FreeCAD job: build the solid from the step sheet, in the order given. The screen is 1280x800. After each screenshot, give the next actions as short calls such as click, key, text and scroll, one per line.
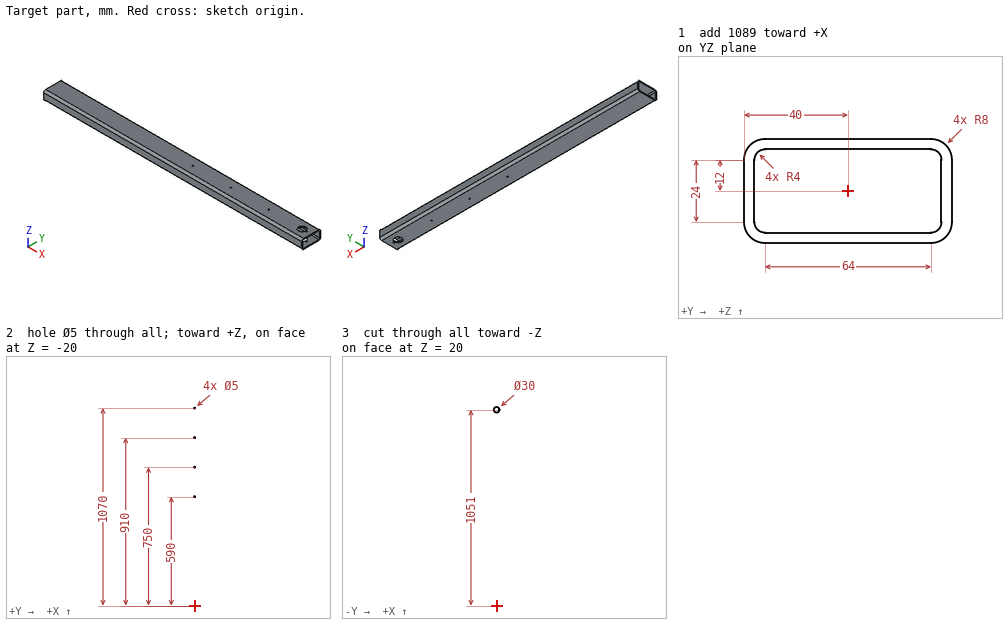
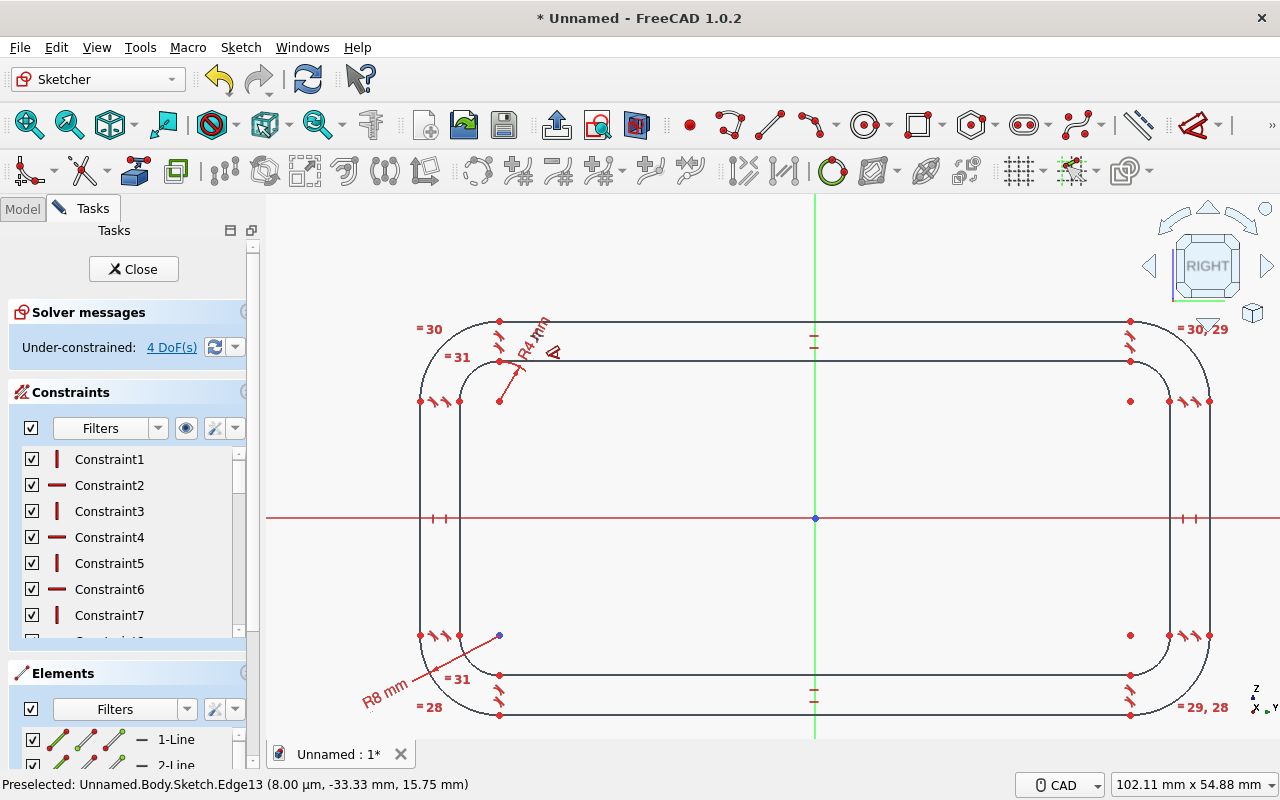
click(420, 471)
click(386, 464)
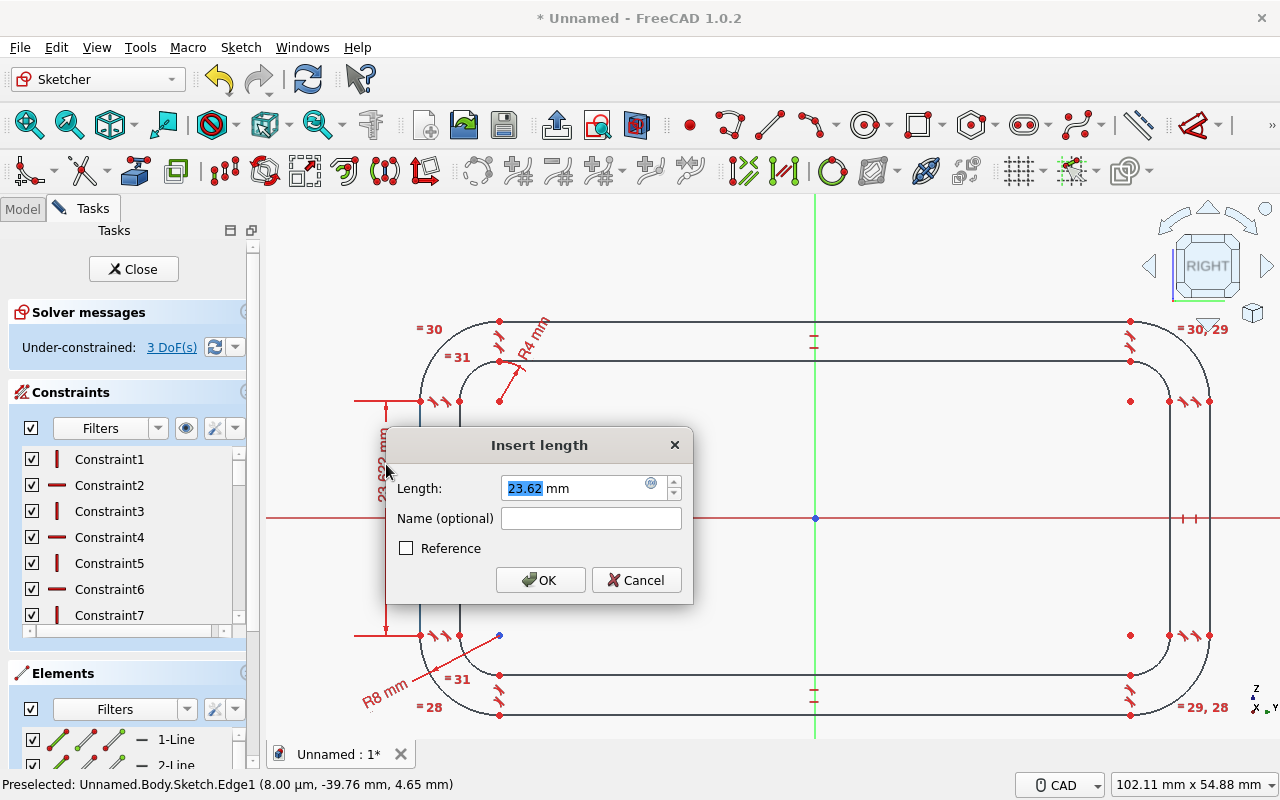
text(24)
key(Return)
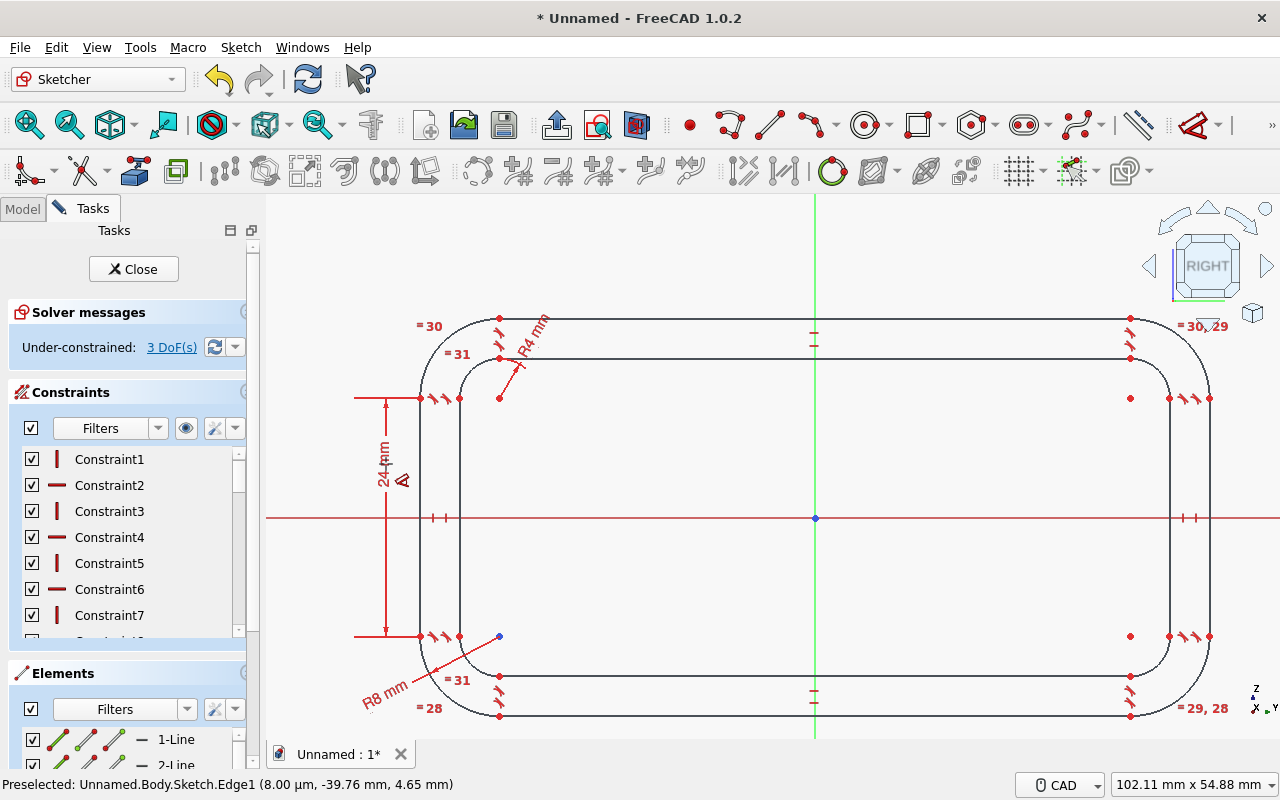
scroll(480, 361, down, 2)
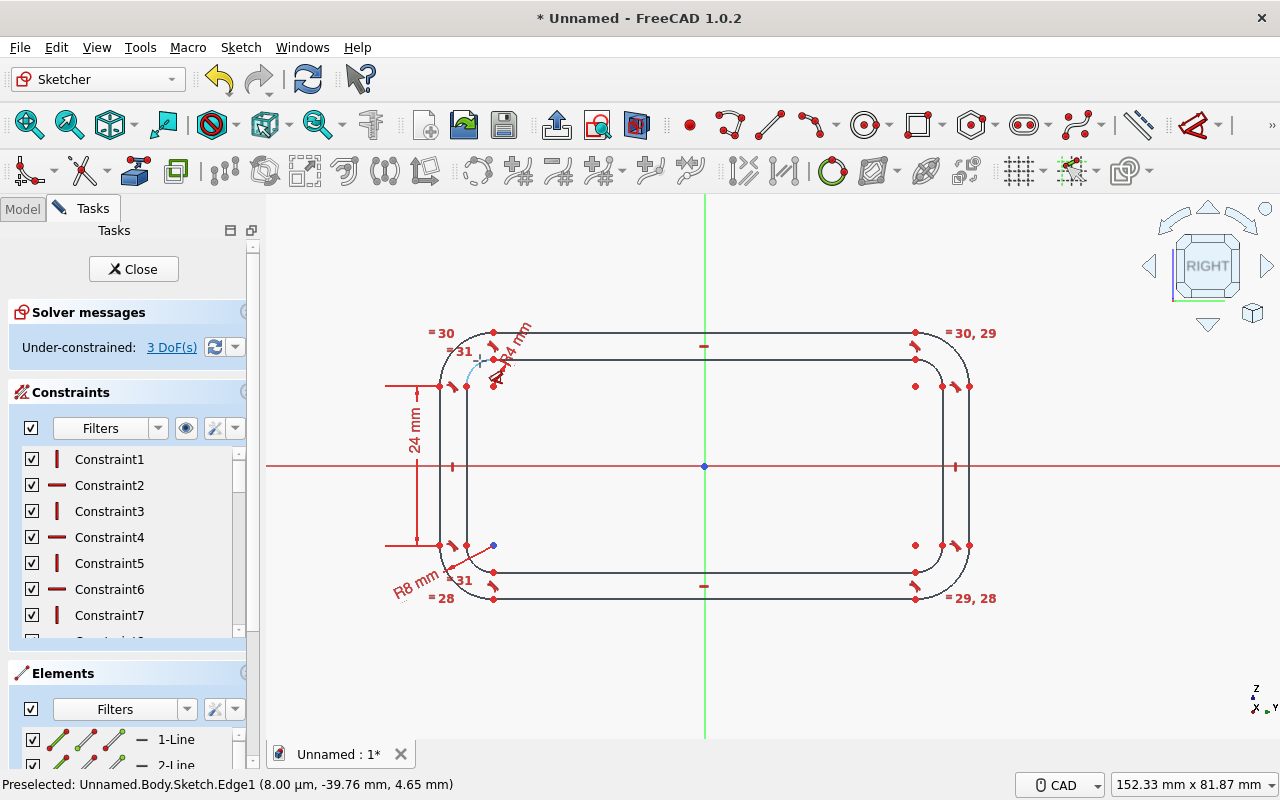
click(620, 599)
click(607, 633)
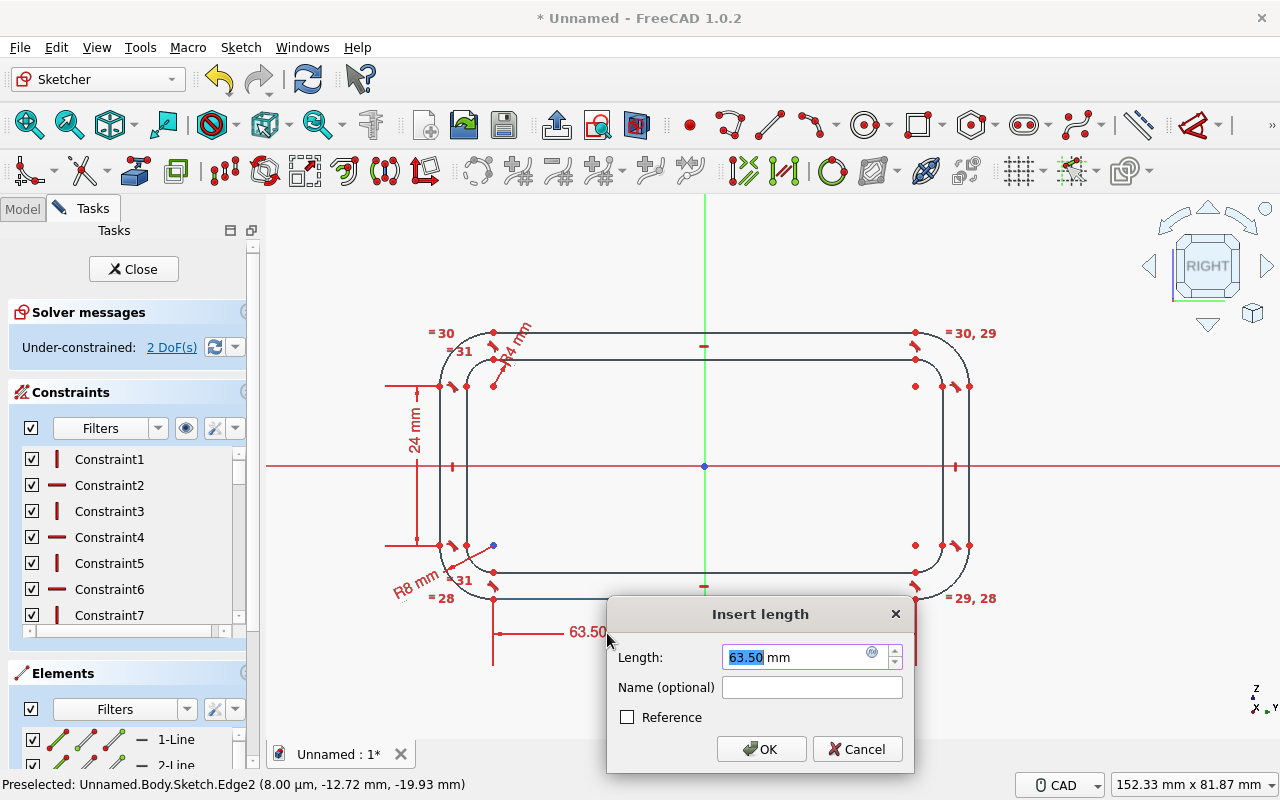
text(64)
key(Return)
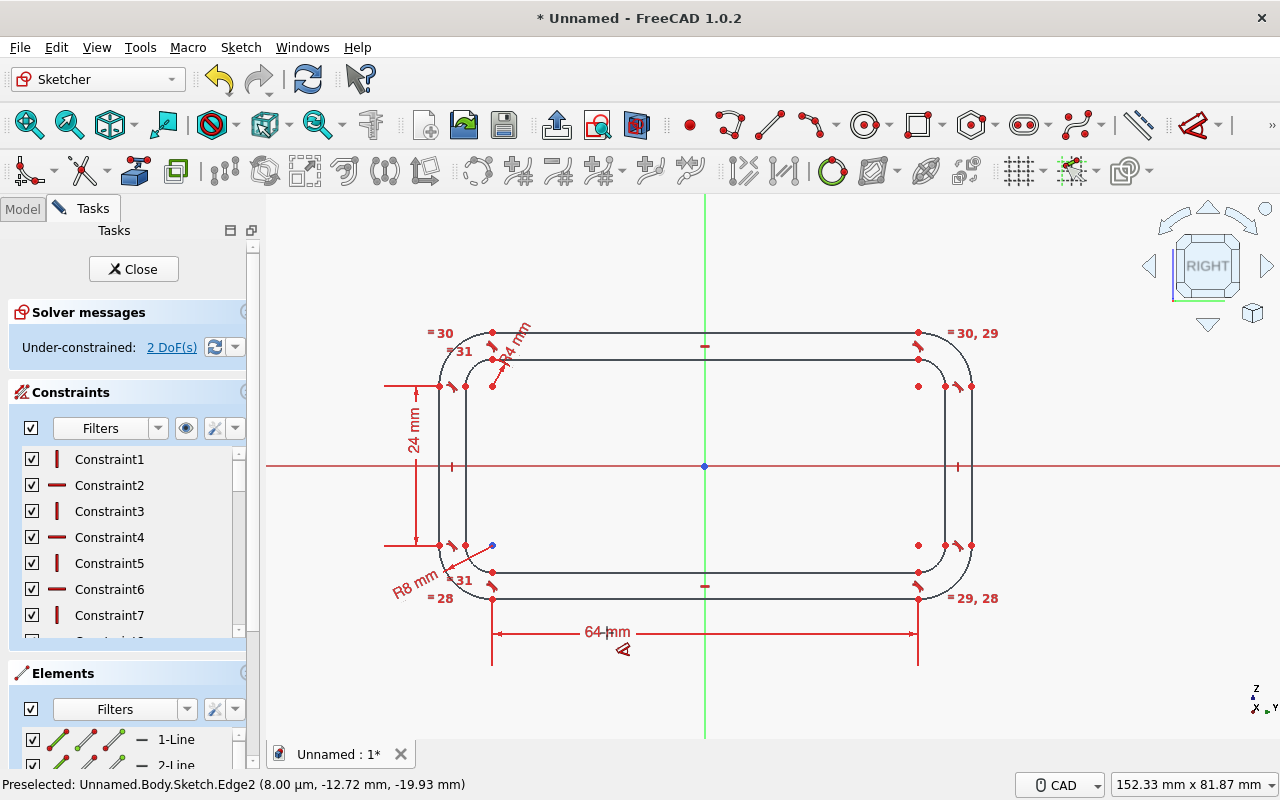
click(439, 386)
click(572, 500)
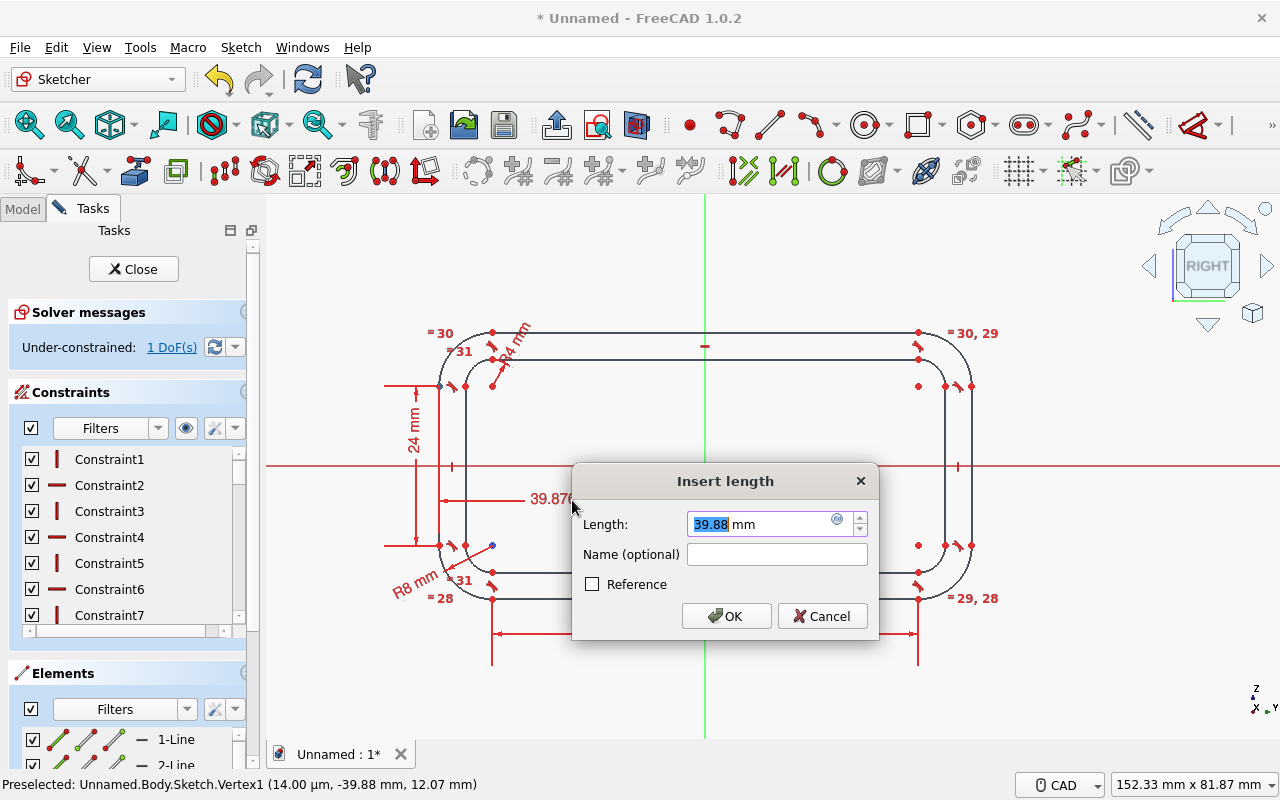
text(40)
key(Return)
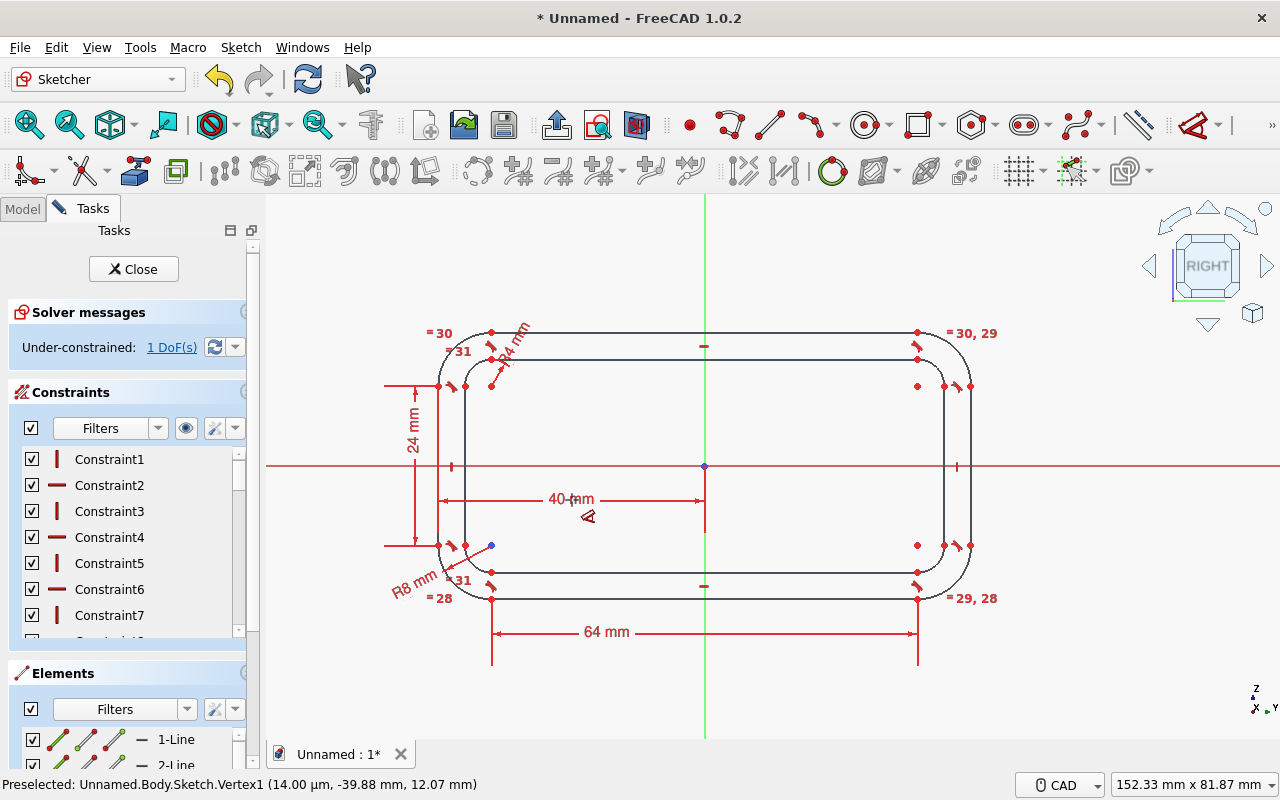
click(438, 386)
click(404, 408)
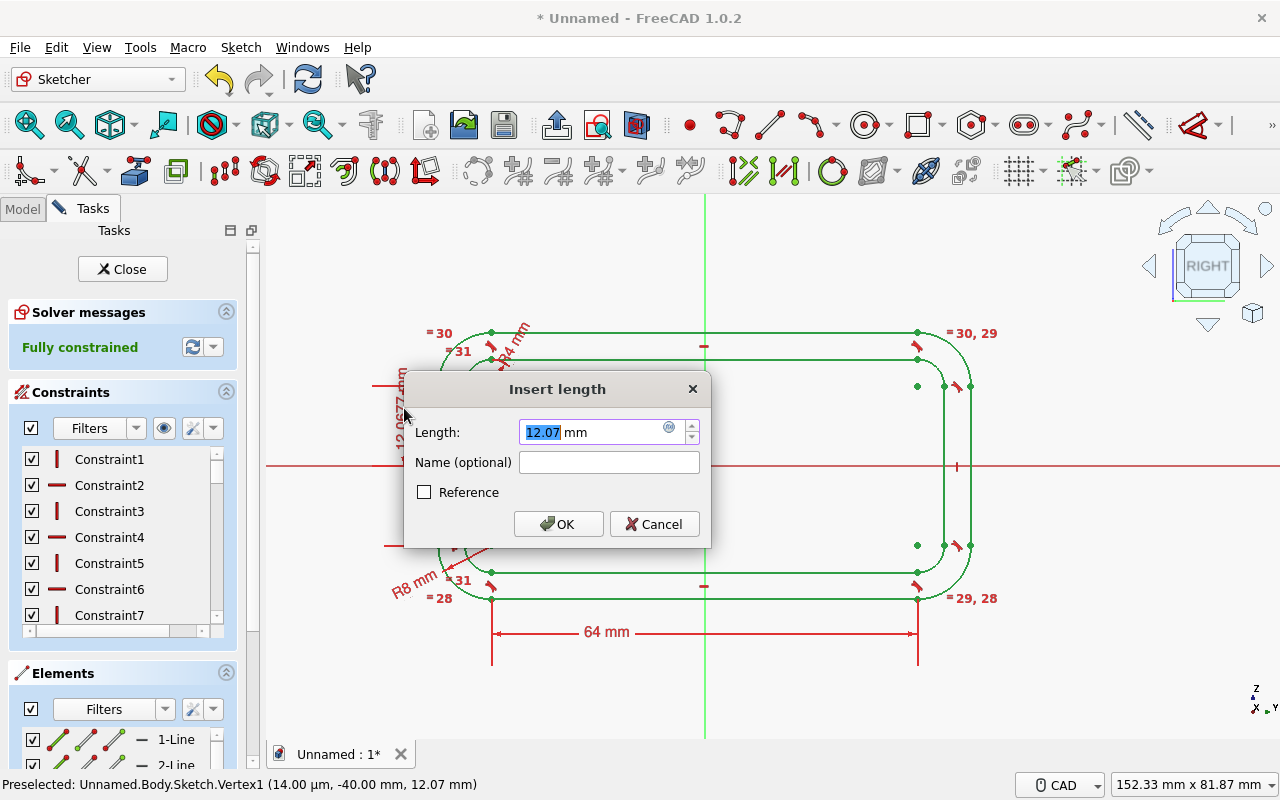
text(12)
key(Return)
key(Escape)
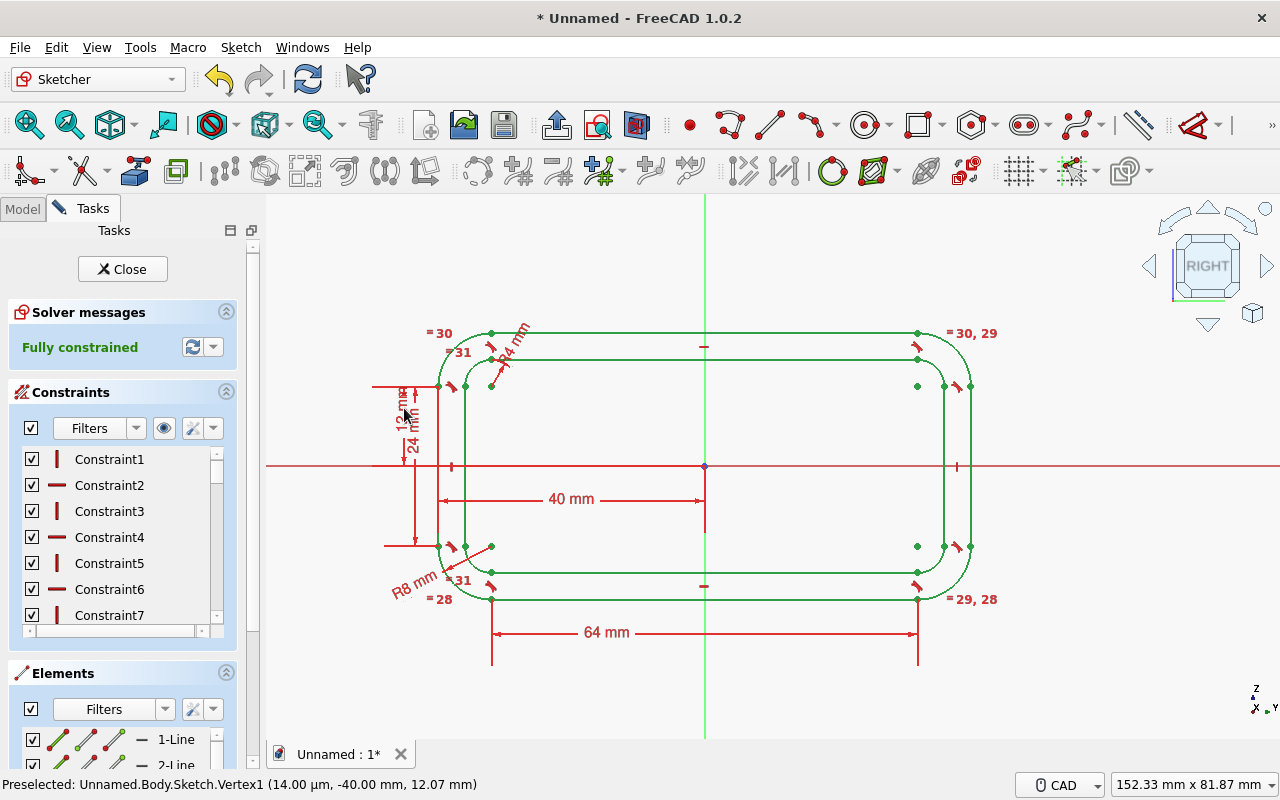
click(123, 269)